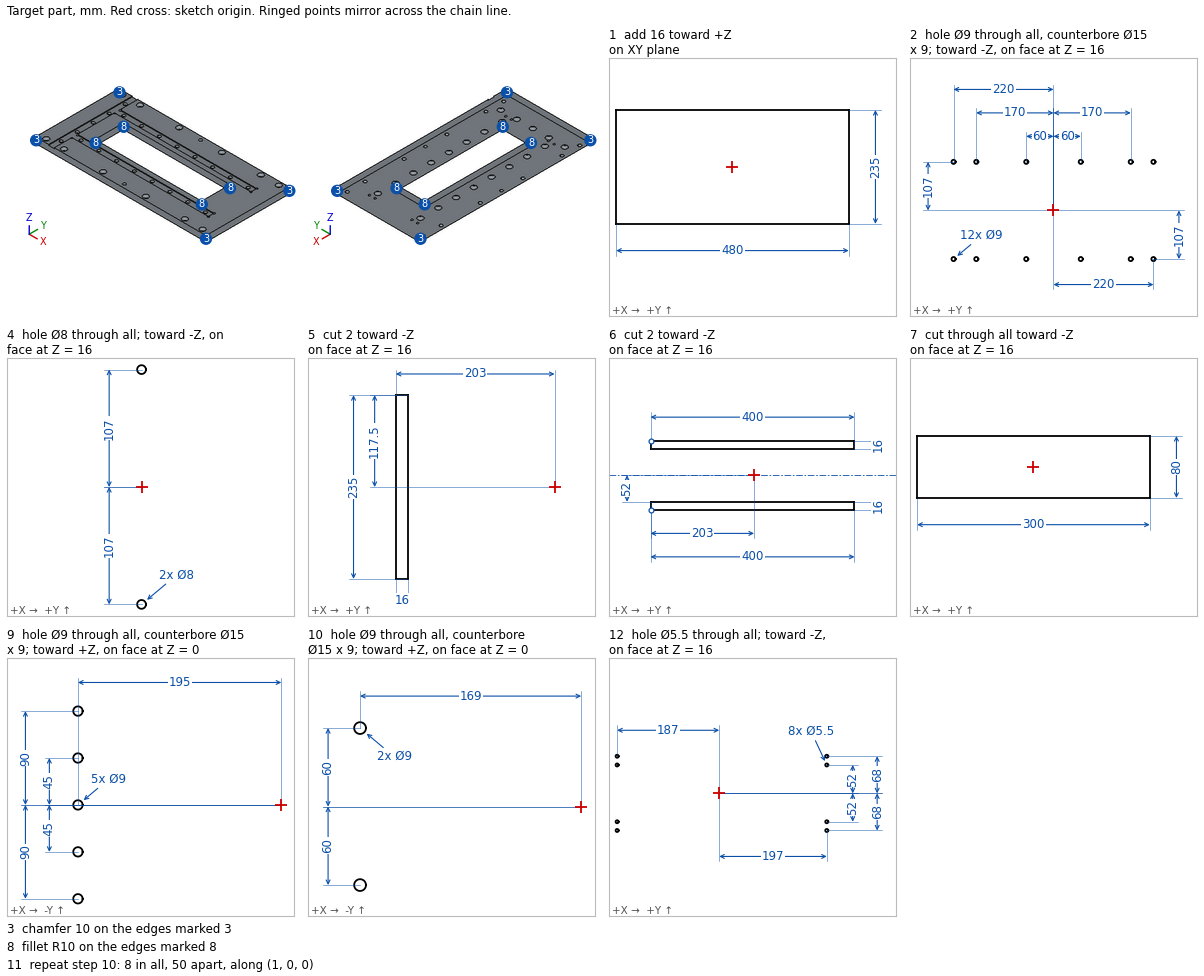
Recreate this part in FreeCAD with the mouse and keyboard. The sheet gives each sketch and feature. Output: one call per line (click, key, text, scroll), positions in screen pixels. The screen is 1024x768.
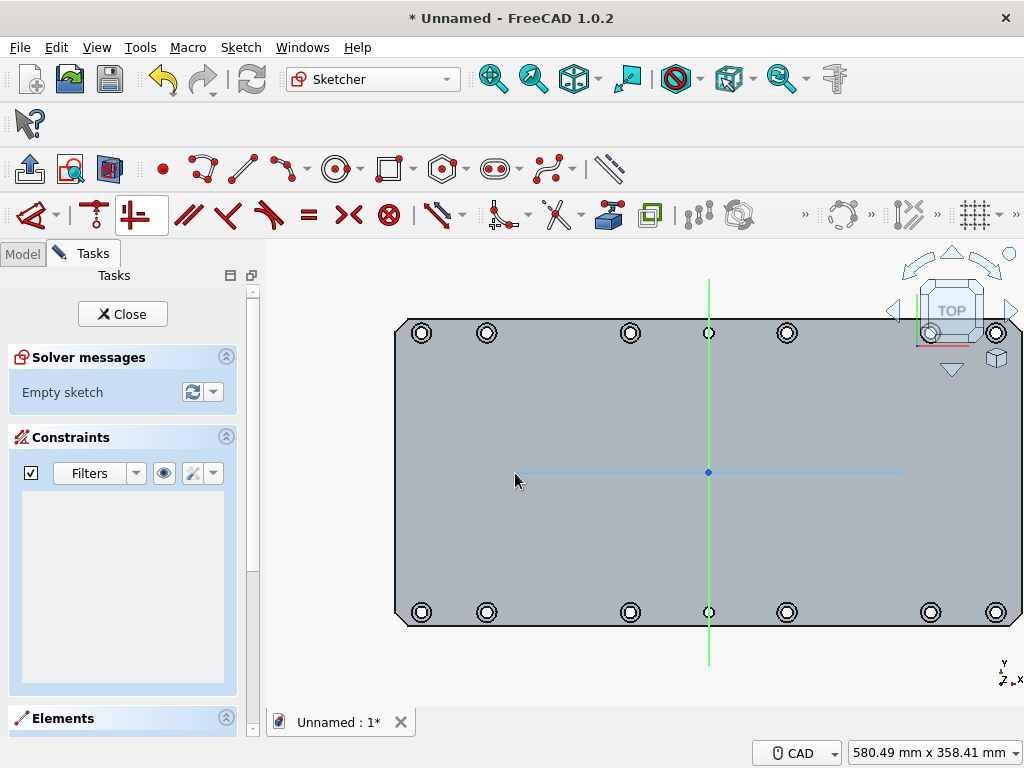
click(390, 170)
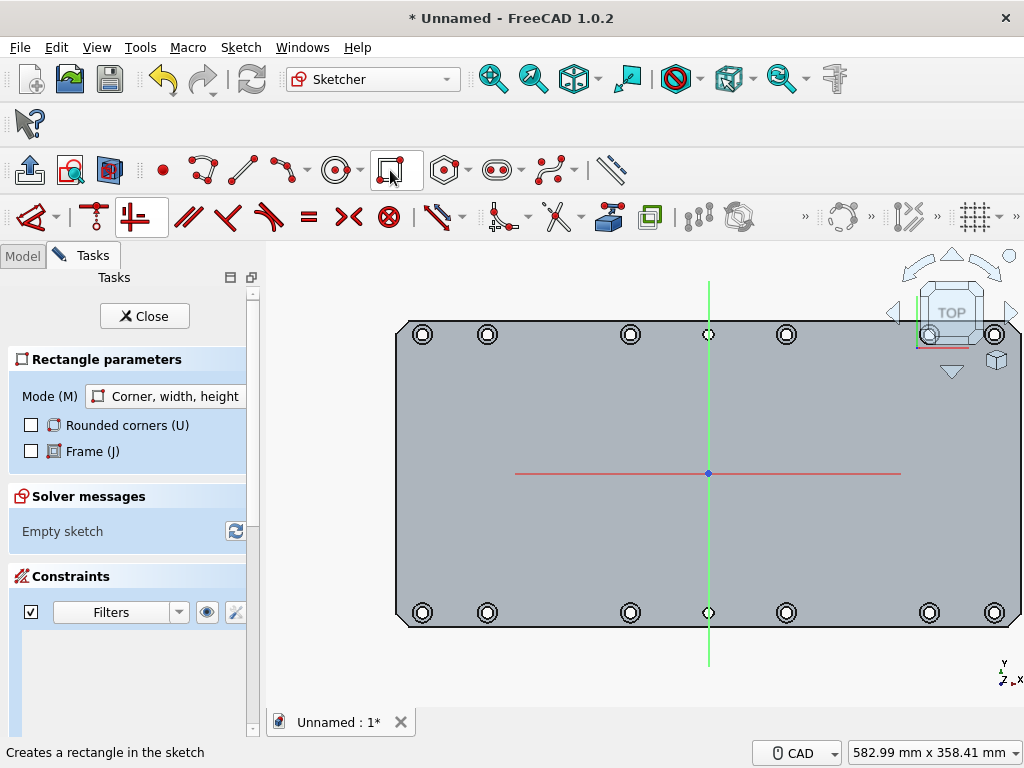
click(445, 321)
move(465, 627)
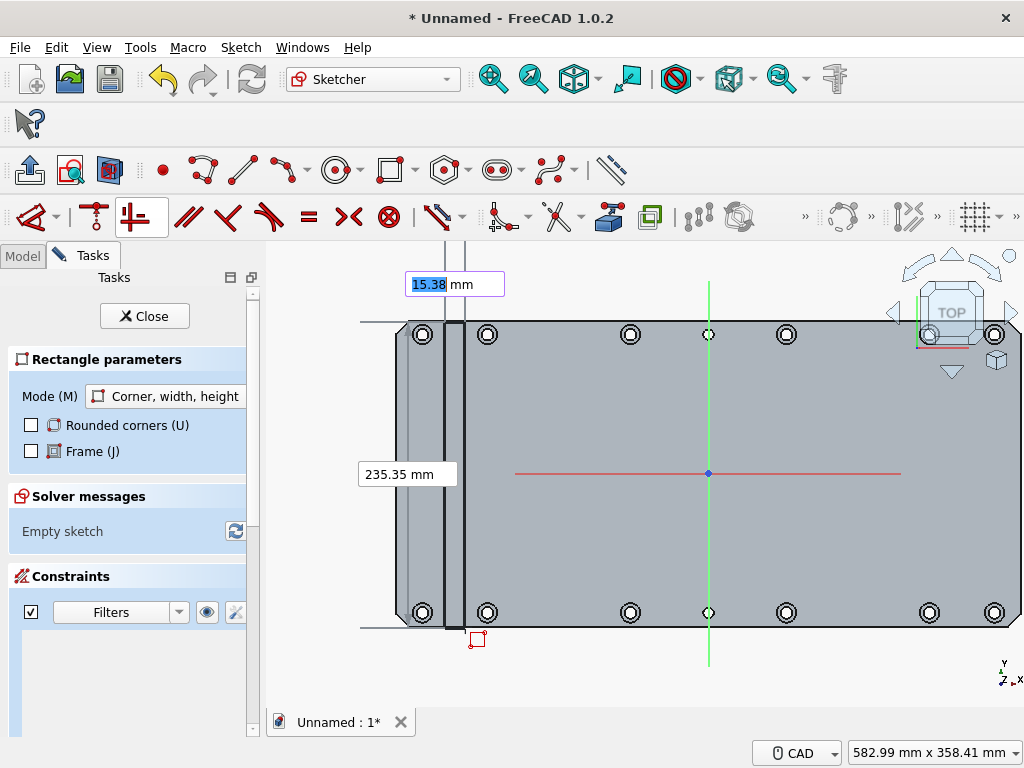
text(16)
key(Tab)
text(235)
key(Return)
key(Escape)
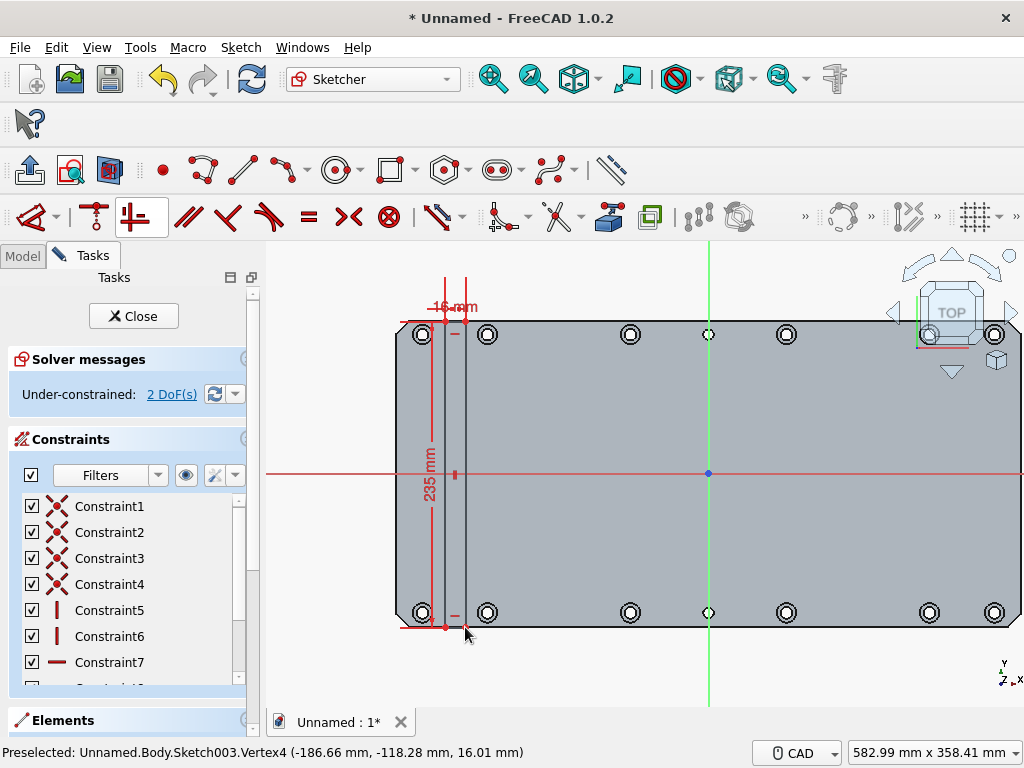
click(32, 218)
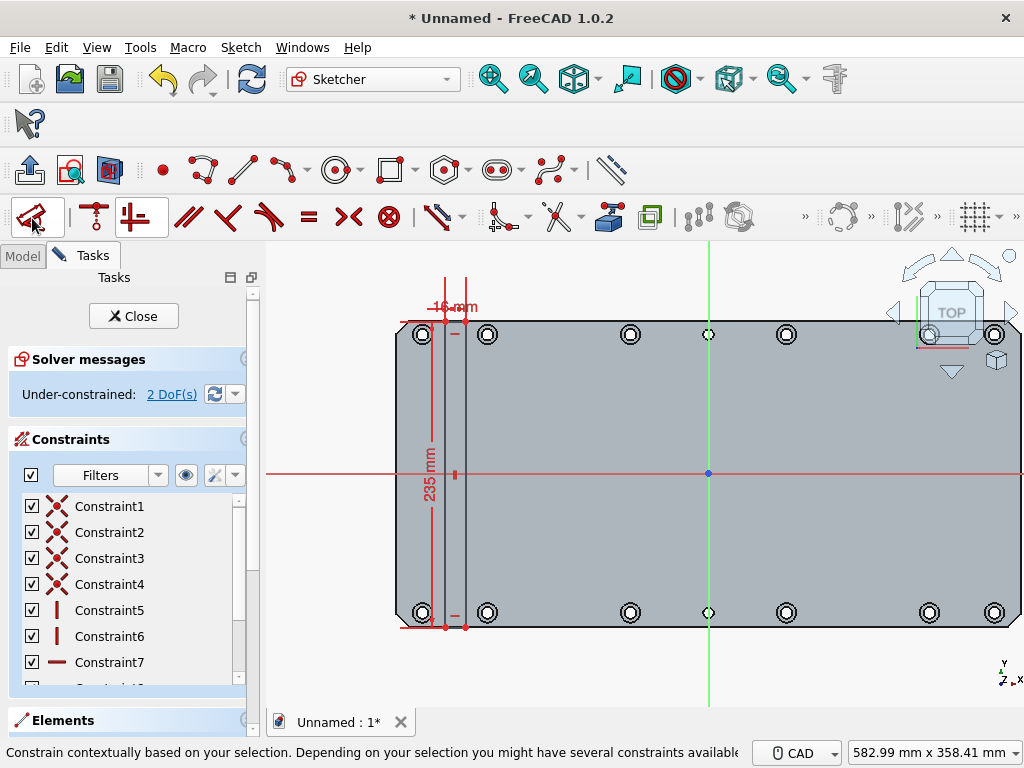
click(445, 322)
click(577, 288)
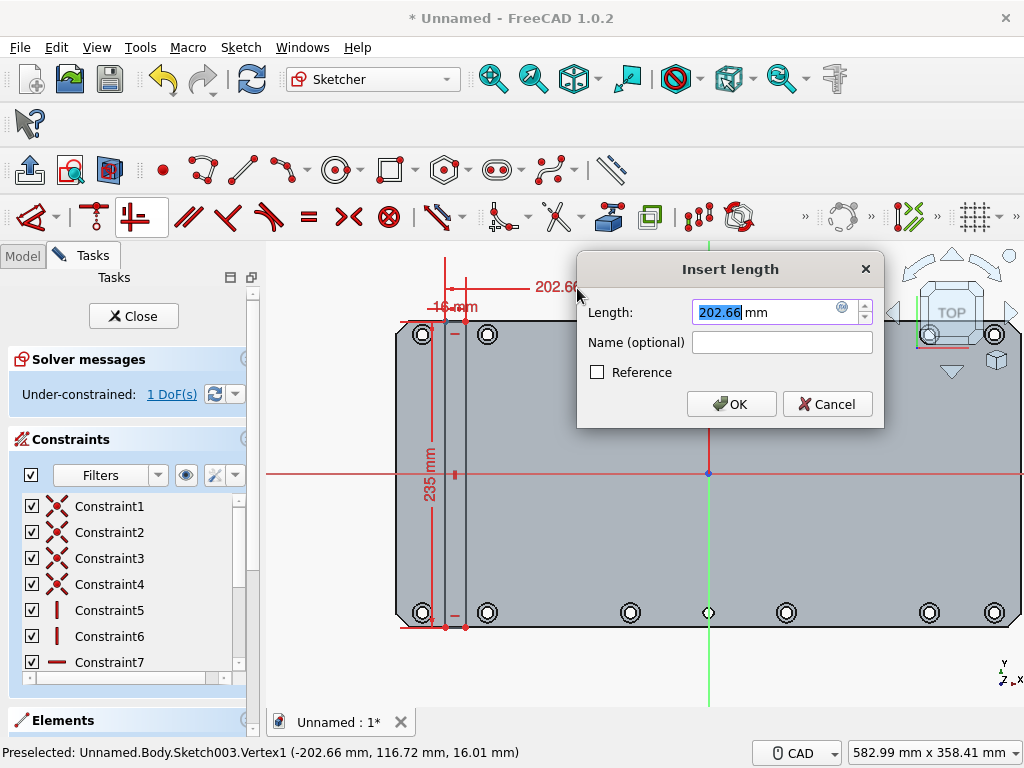
text(203)
key(Return)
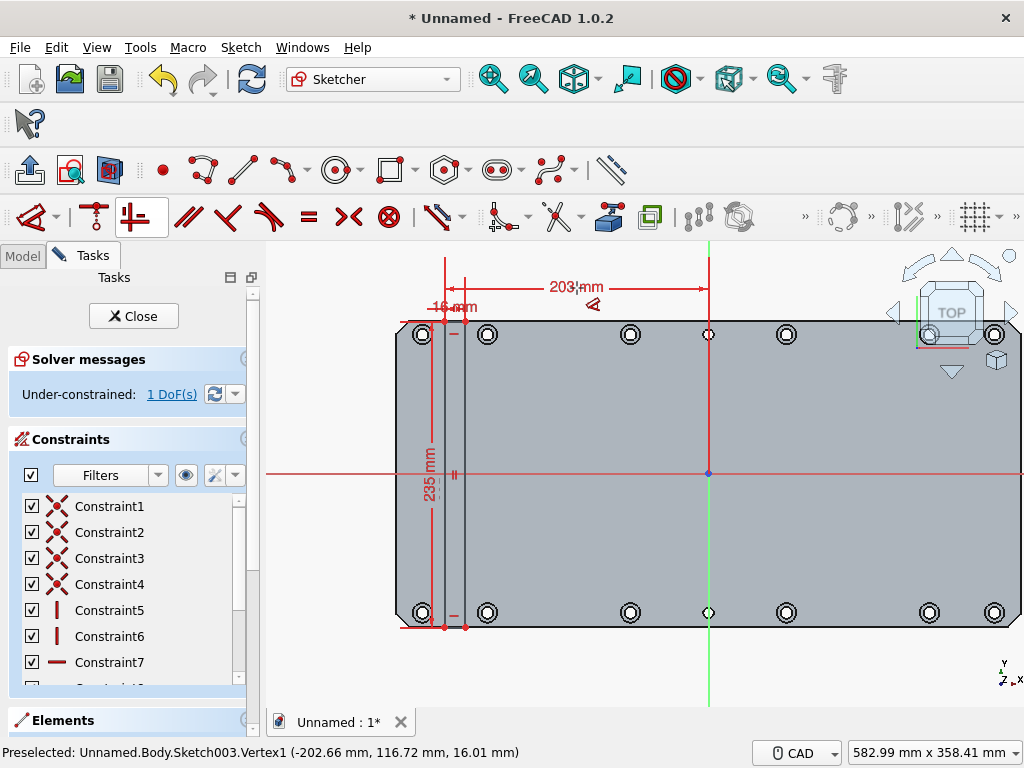
click(445, 322)
click(743, 398)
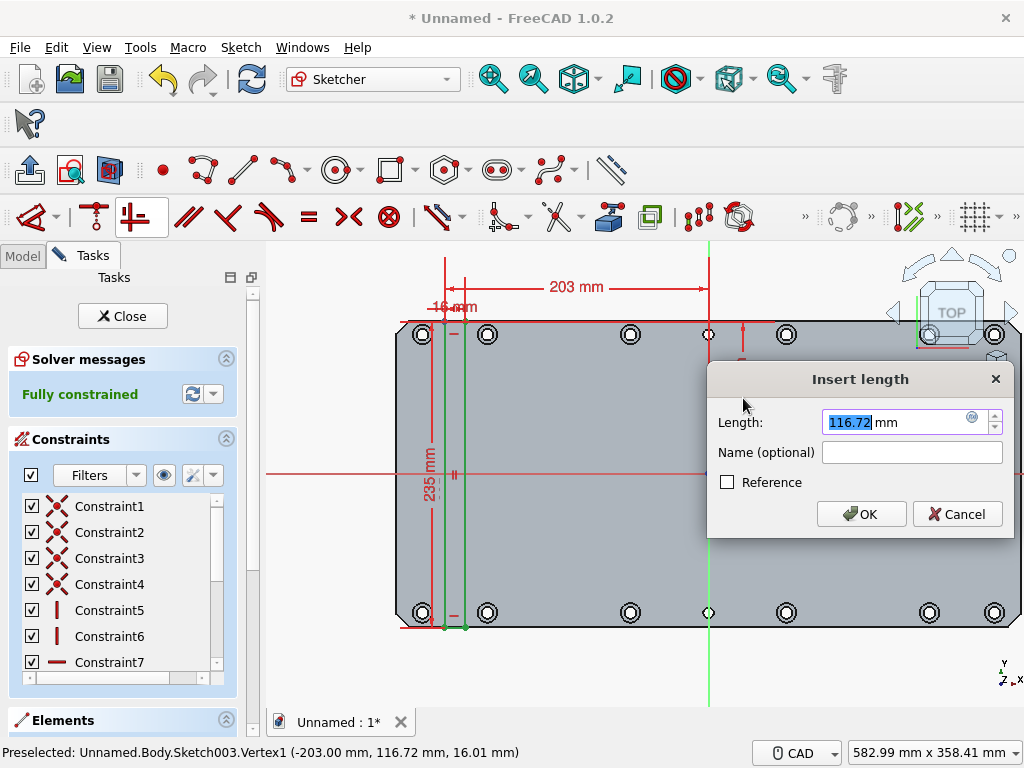
text(117.5)
key(Return)
key(Escape)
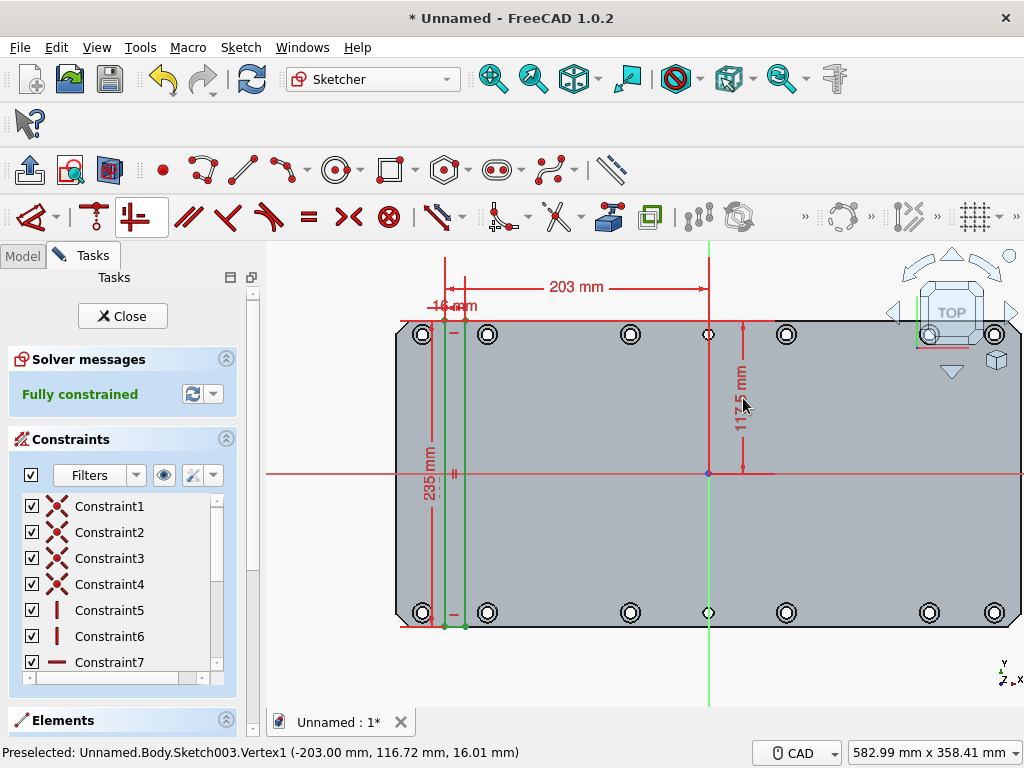
click(123, 316)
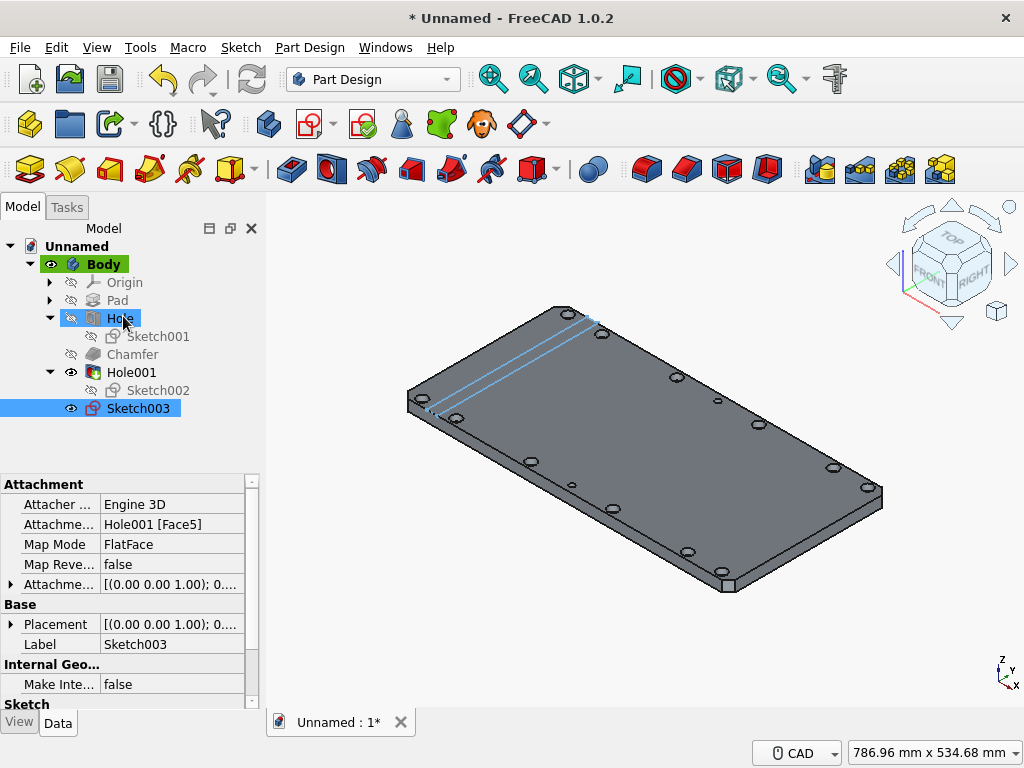
click(292, 170)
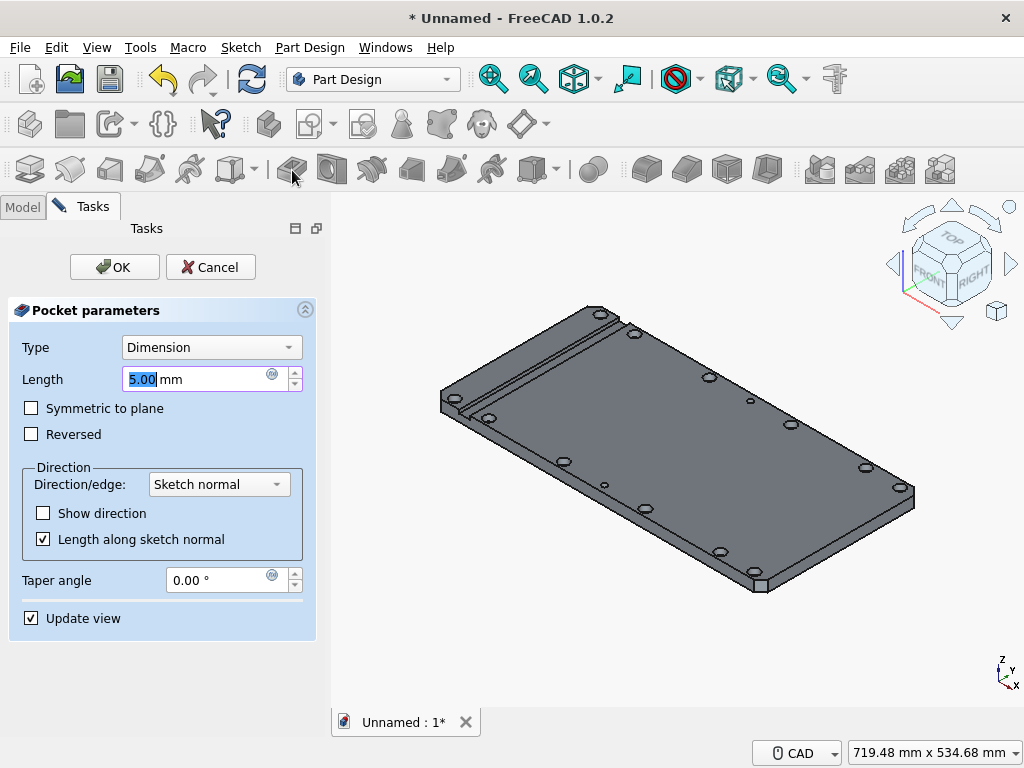
text(2)
key(Tab)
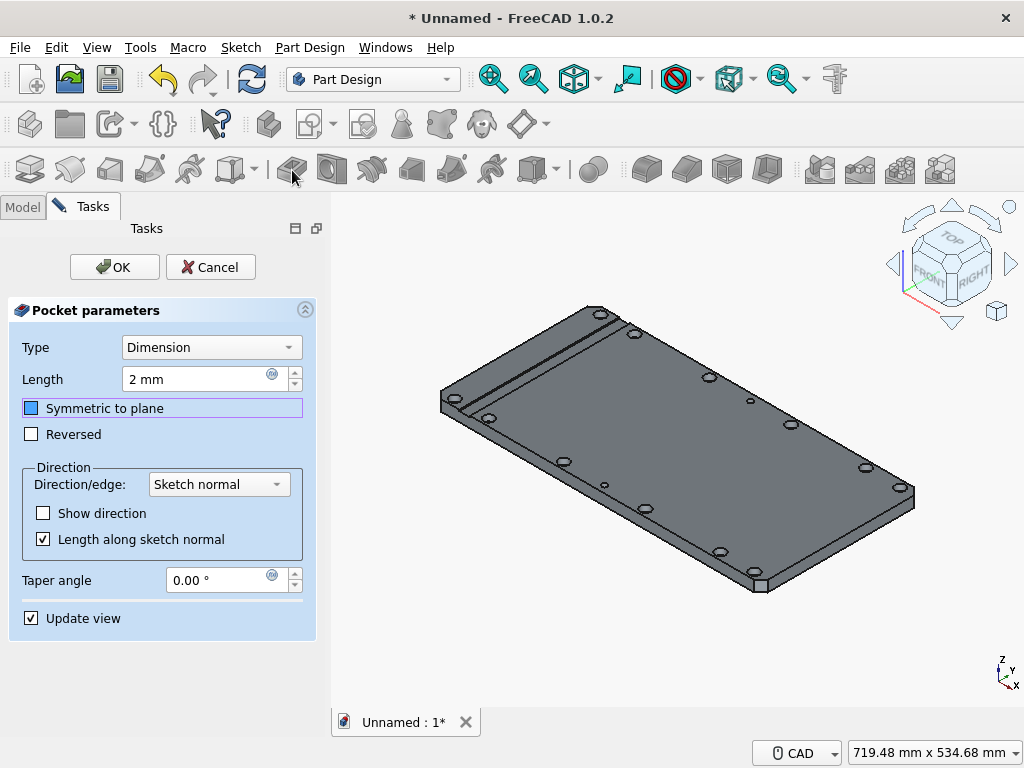
click(115, 267)